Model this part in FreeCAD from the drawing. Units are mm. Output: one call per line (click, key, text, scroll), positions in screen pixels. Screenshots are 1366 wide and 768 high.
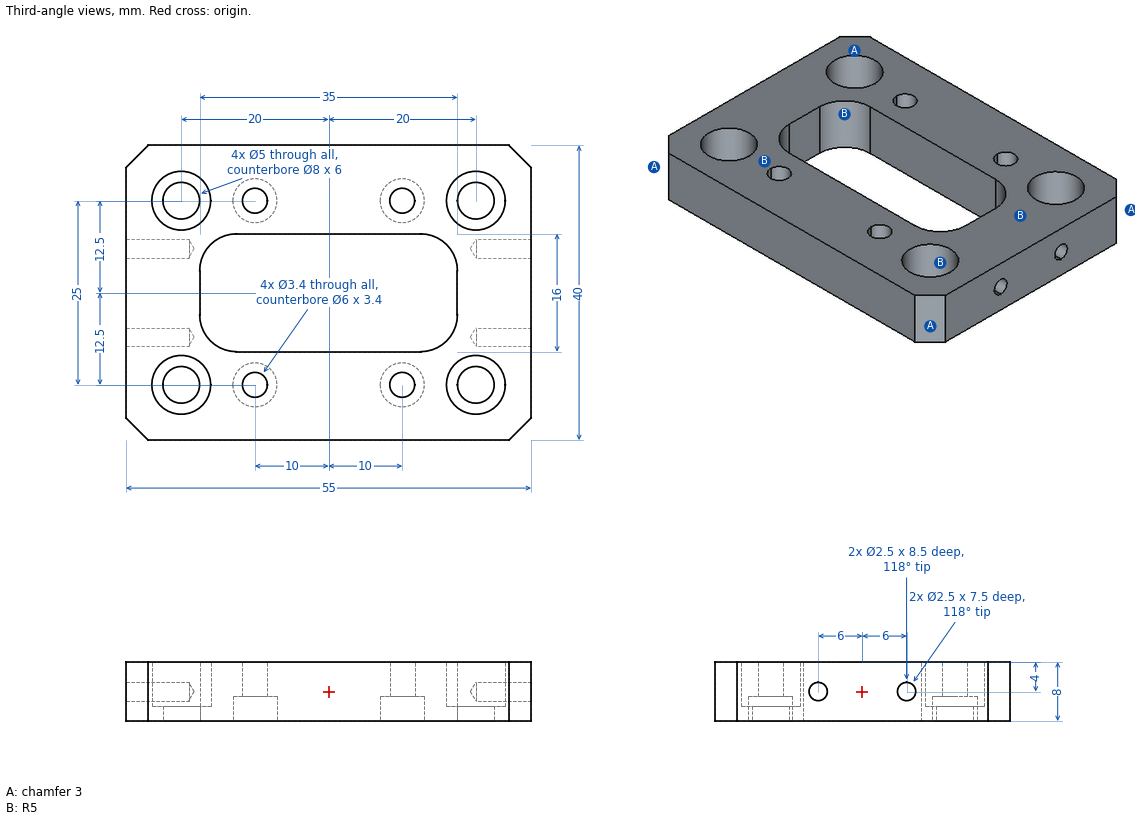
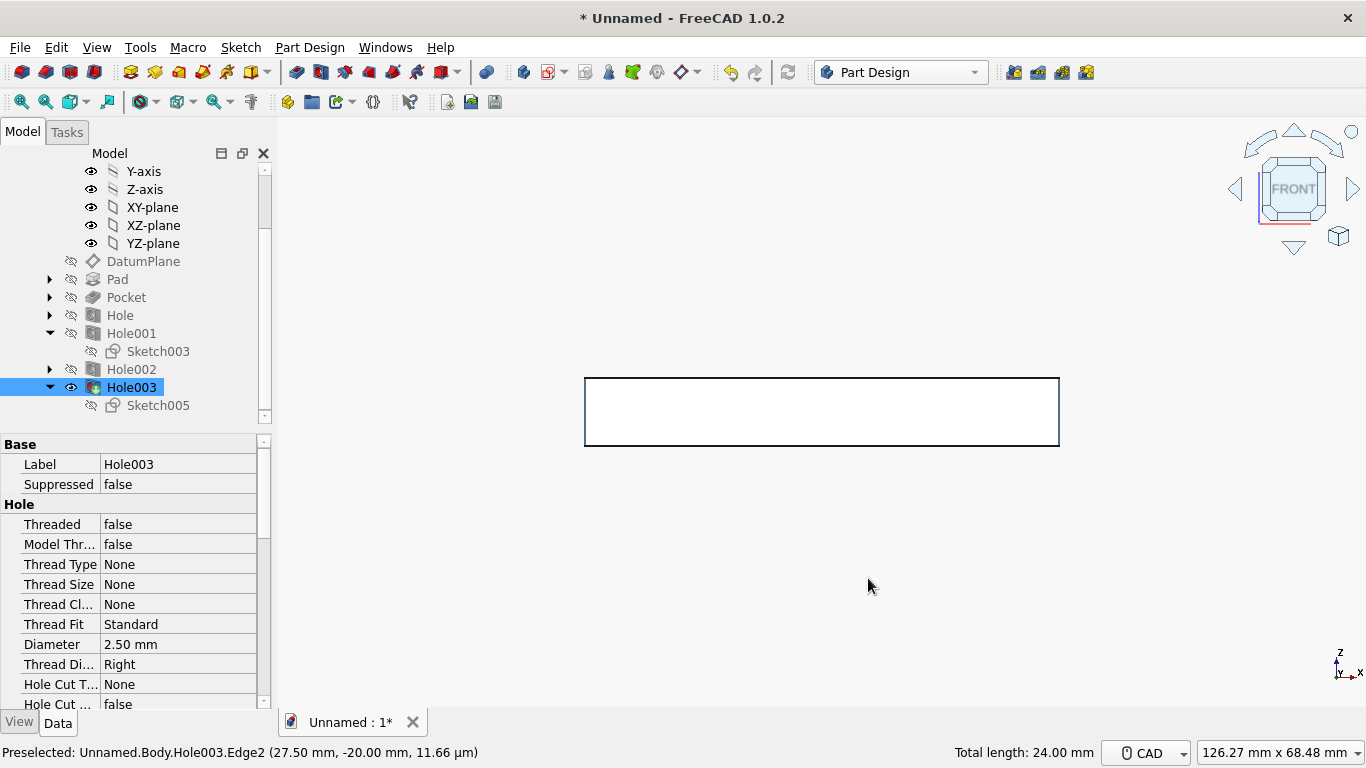
click(22, 102)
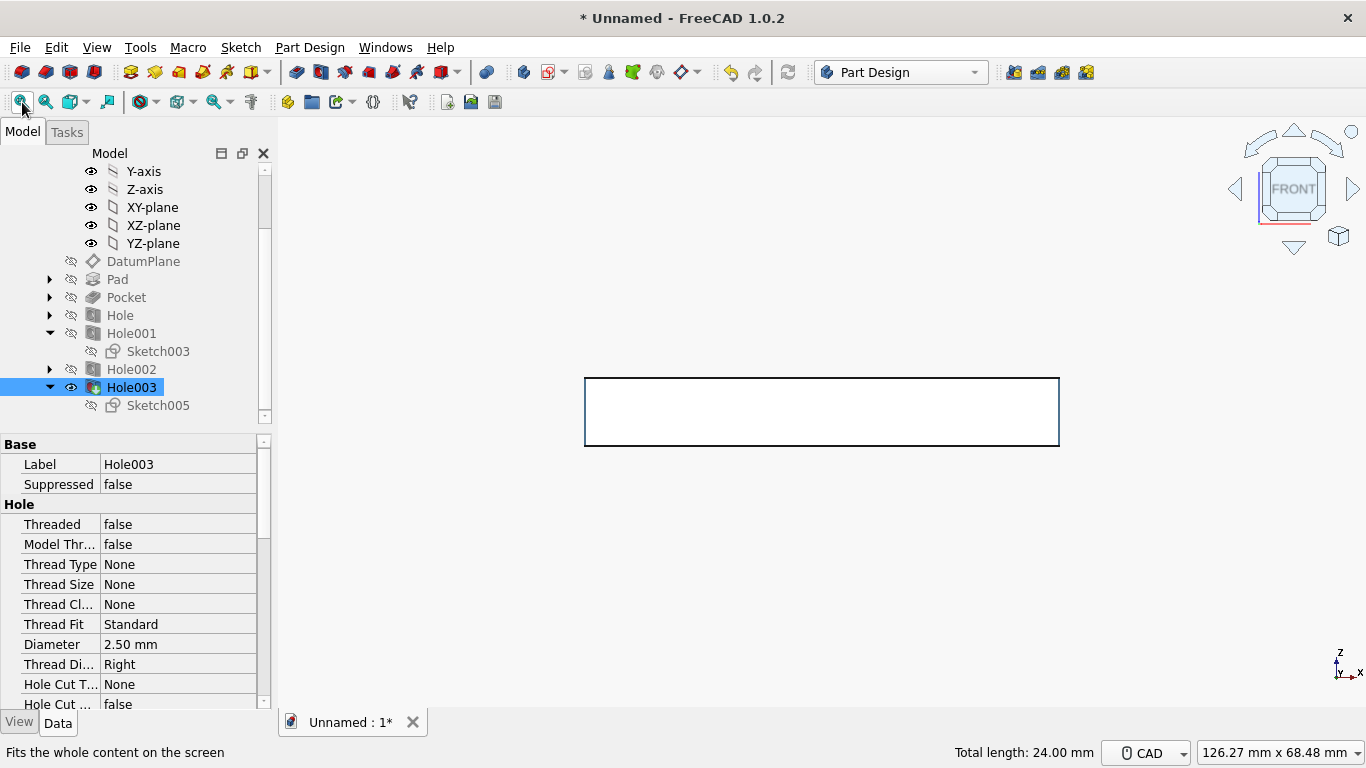
key(3)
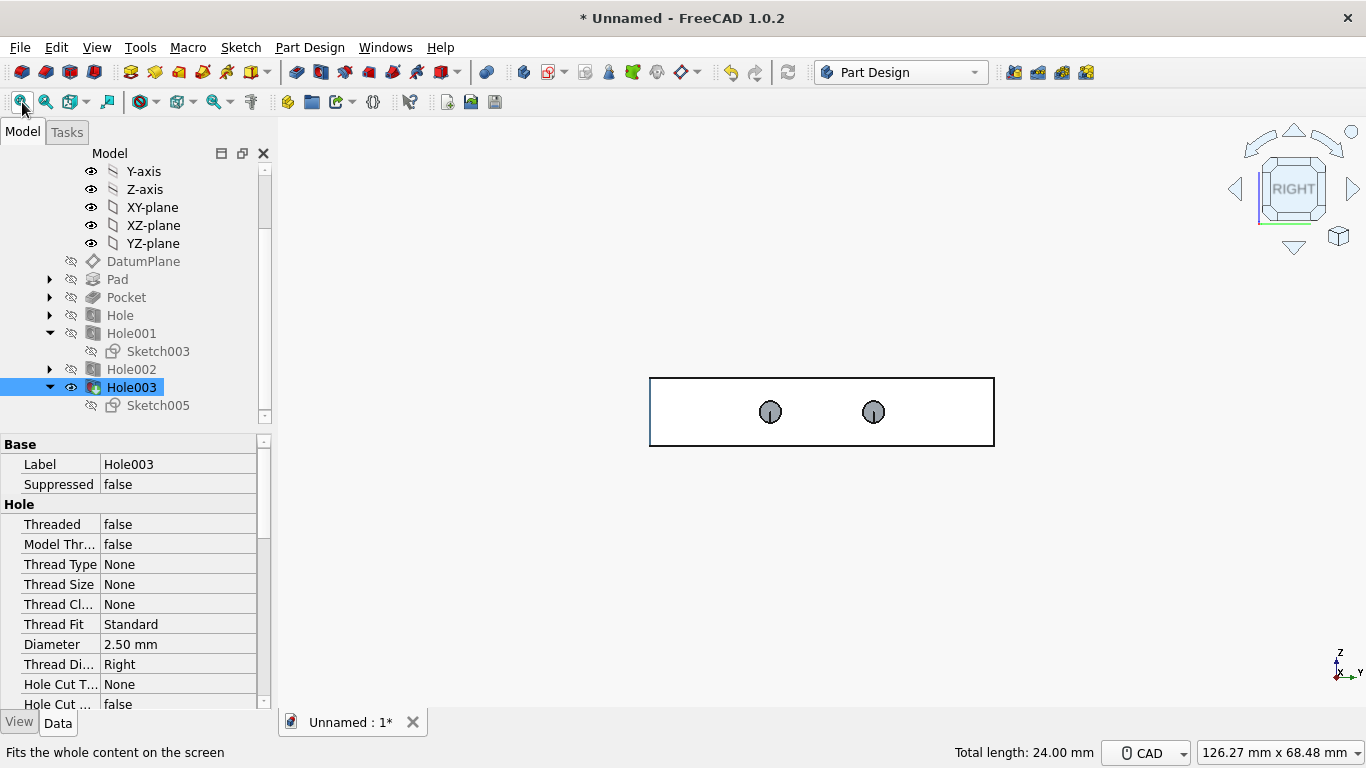
click(22, 102)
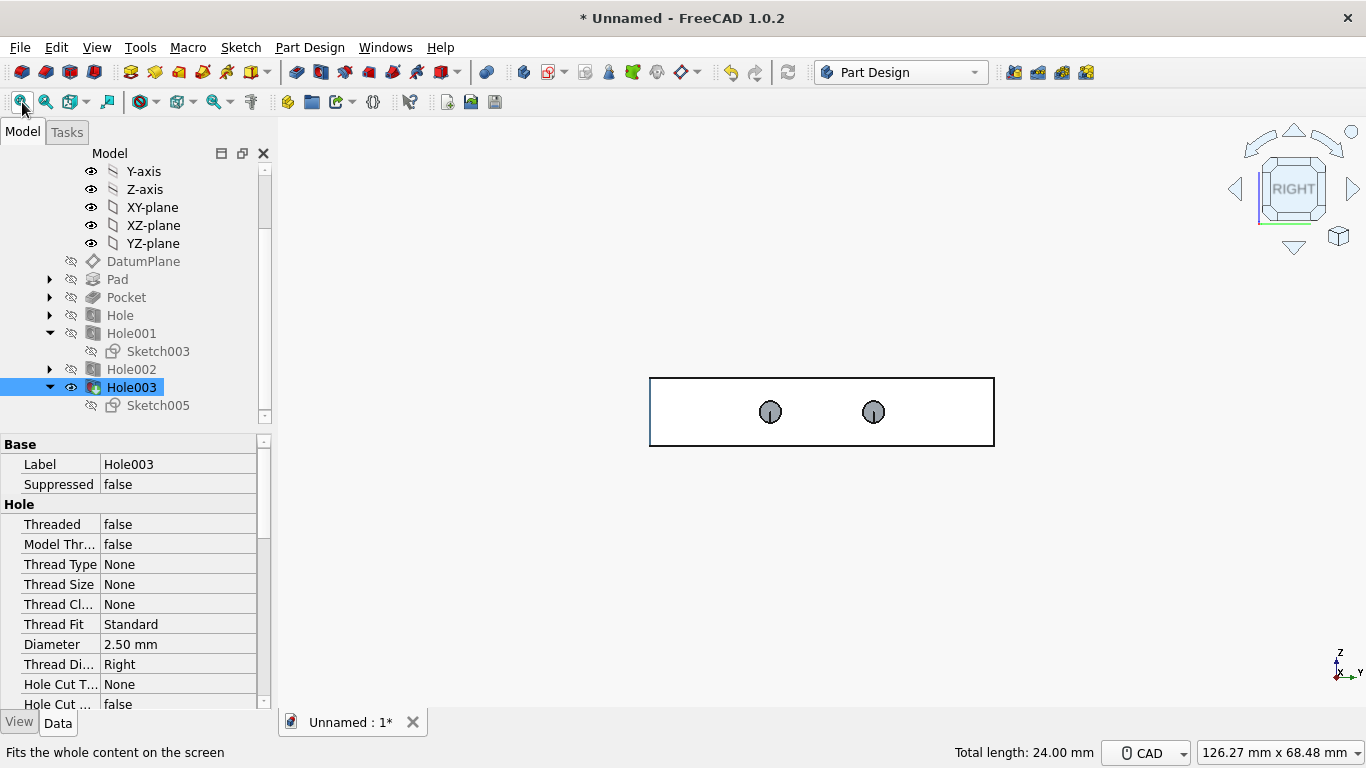
click(994, 411, ctrl)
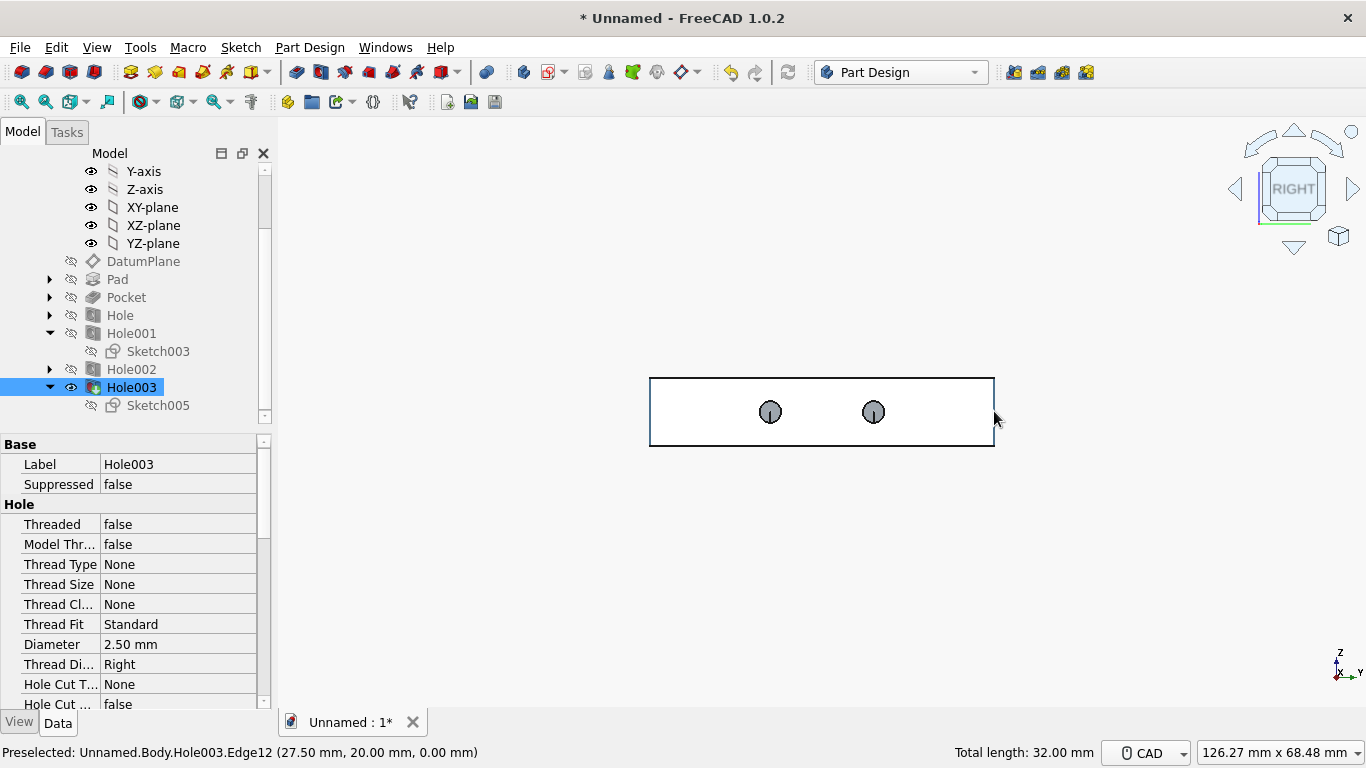
click(46, 72)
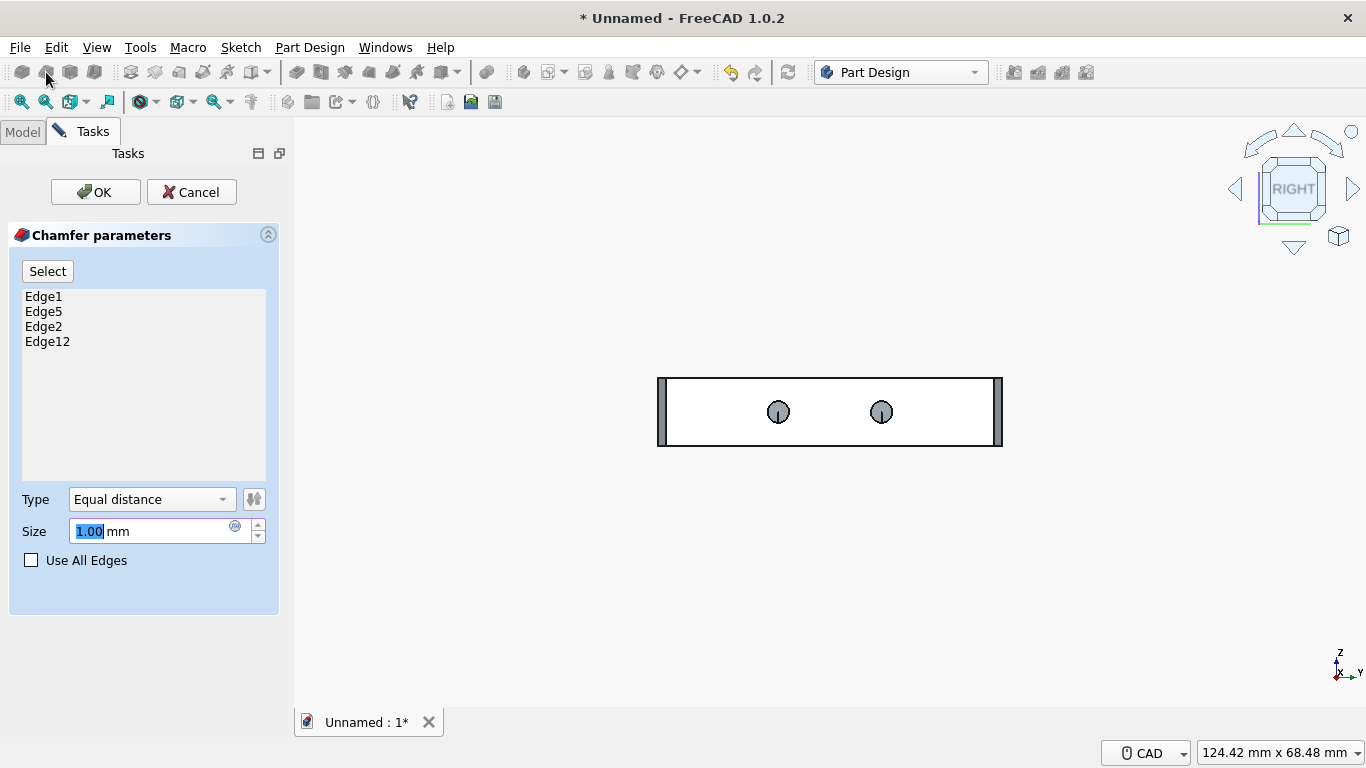
text(3)
key(Tab)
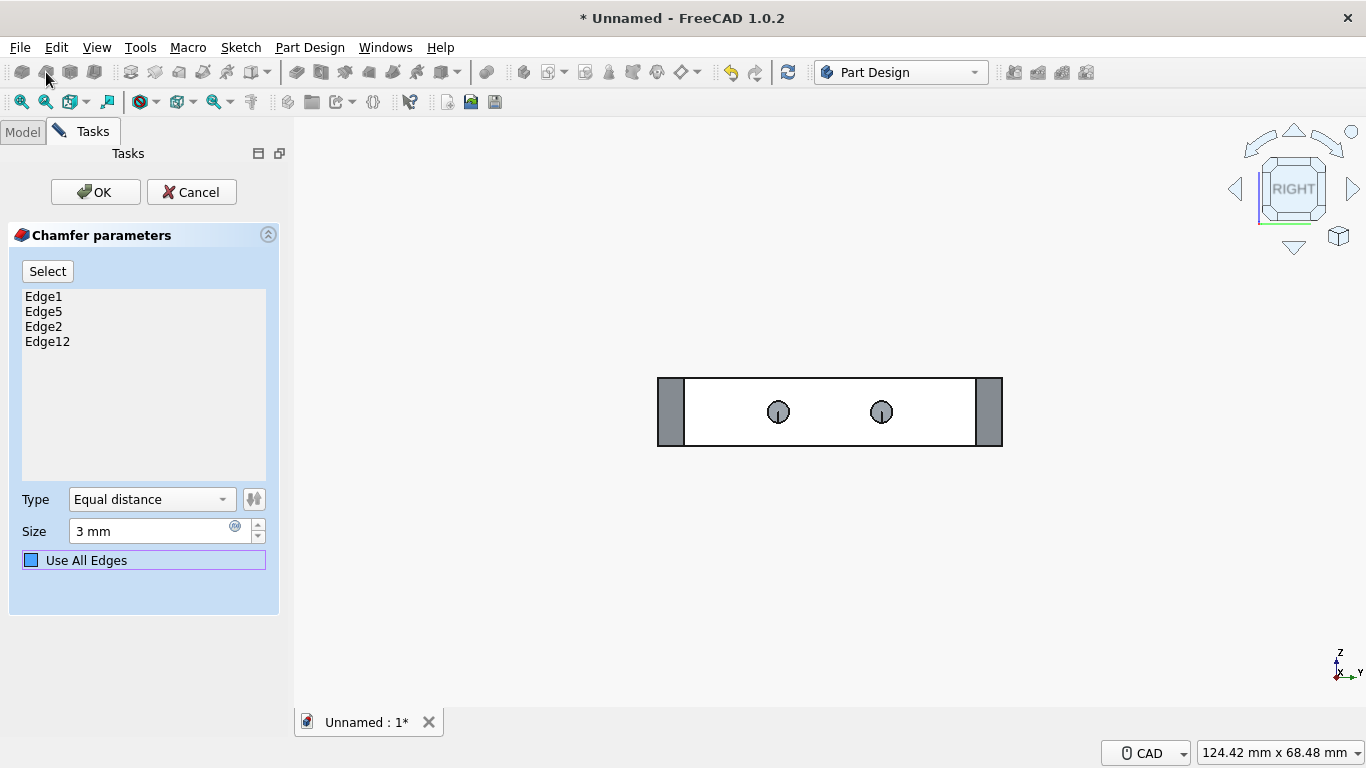
click(96, 192)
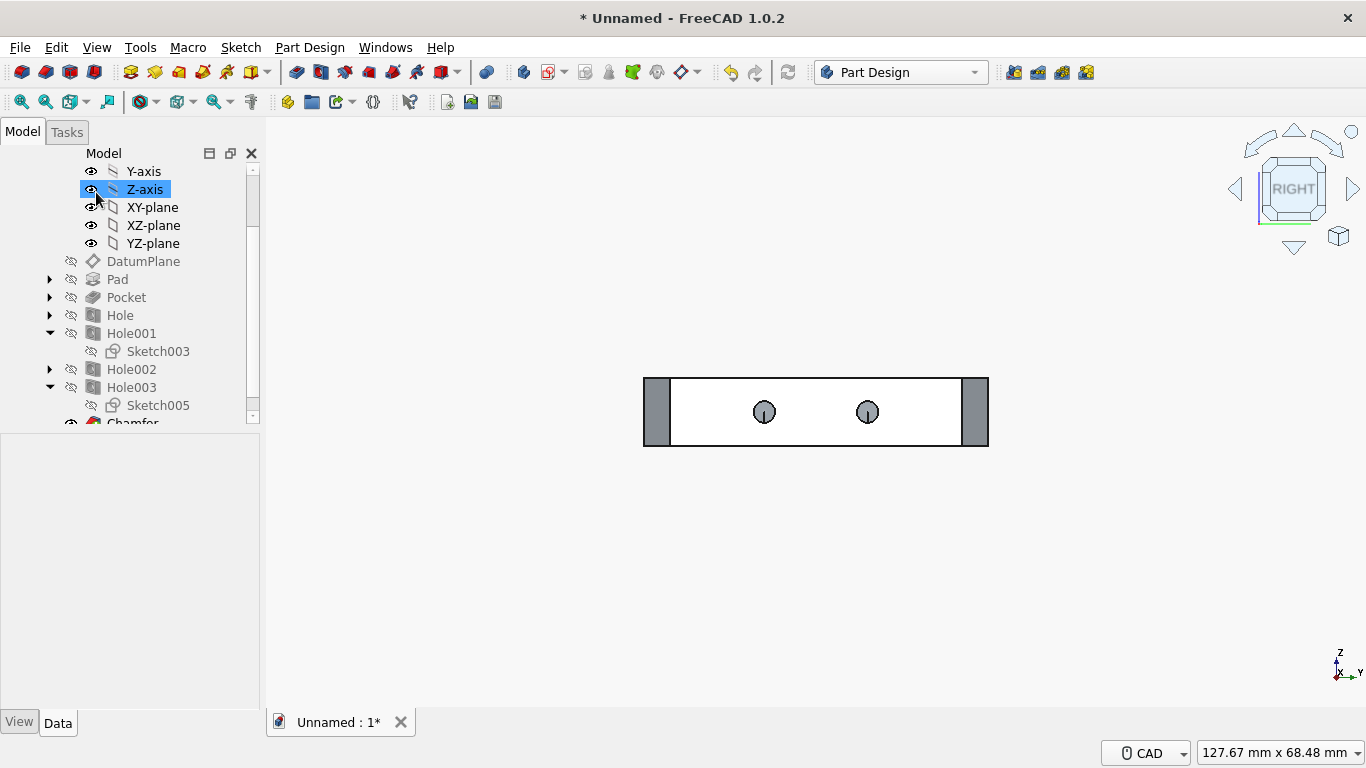
click(22, 102)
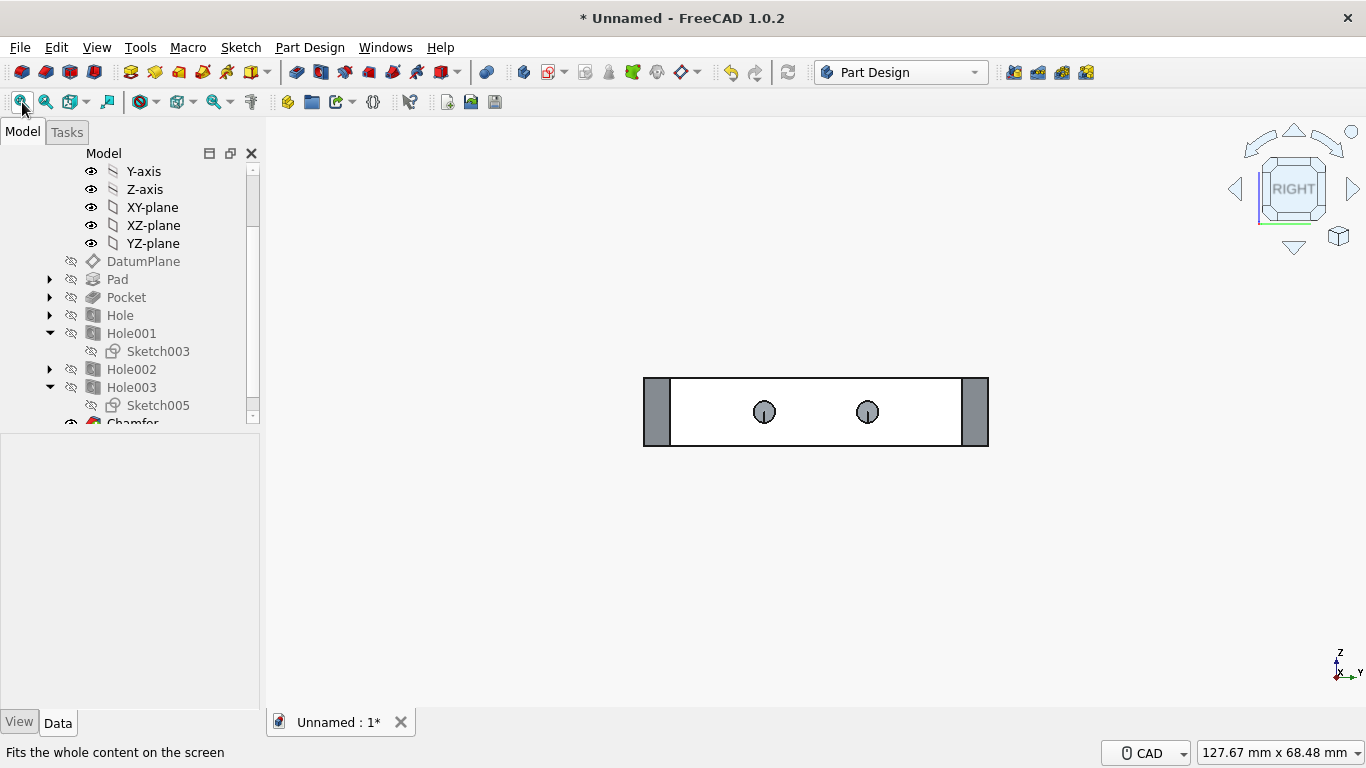
key(0)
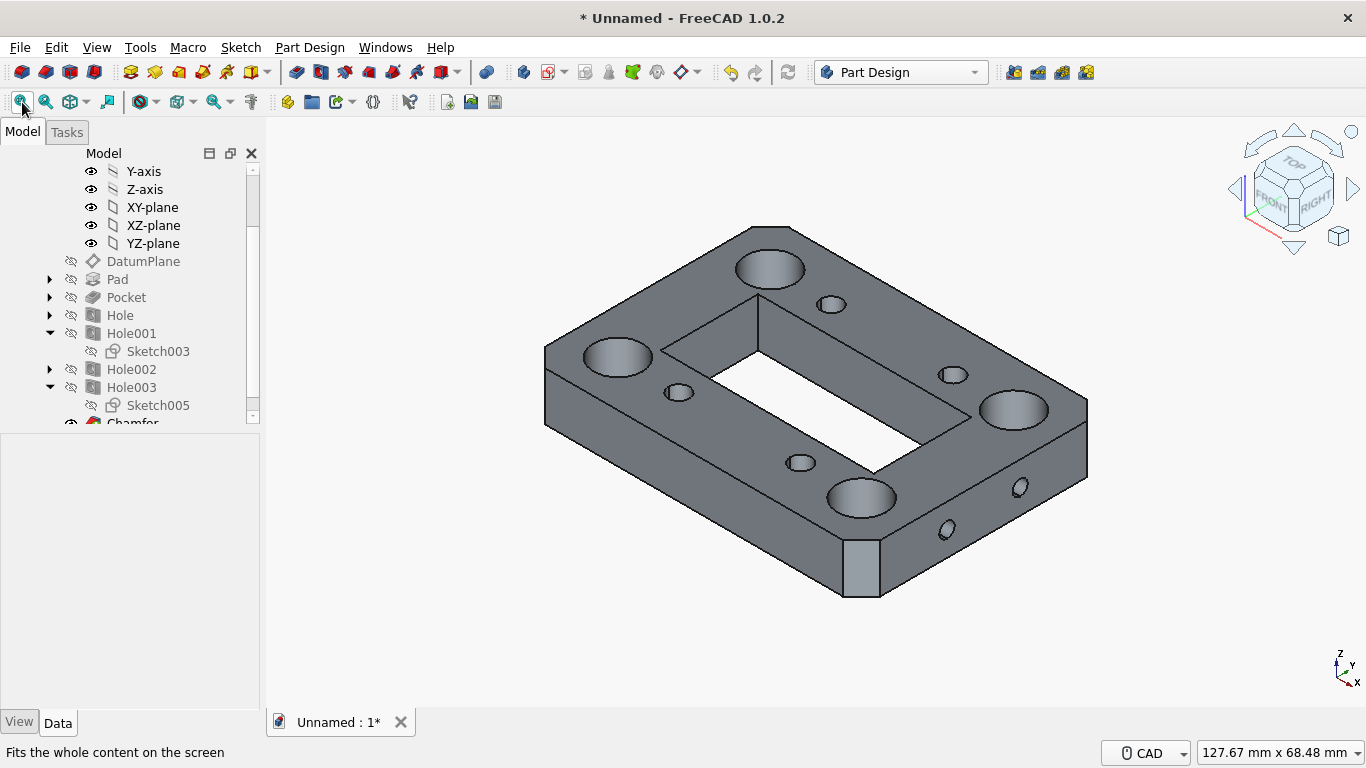
key(2)